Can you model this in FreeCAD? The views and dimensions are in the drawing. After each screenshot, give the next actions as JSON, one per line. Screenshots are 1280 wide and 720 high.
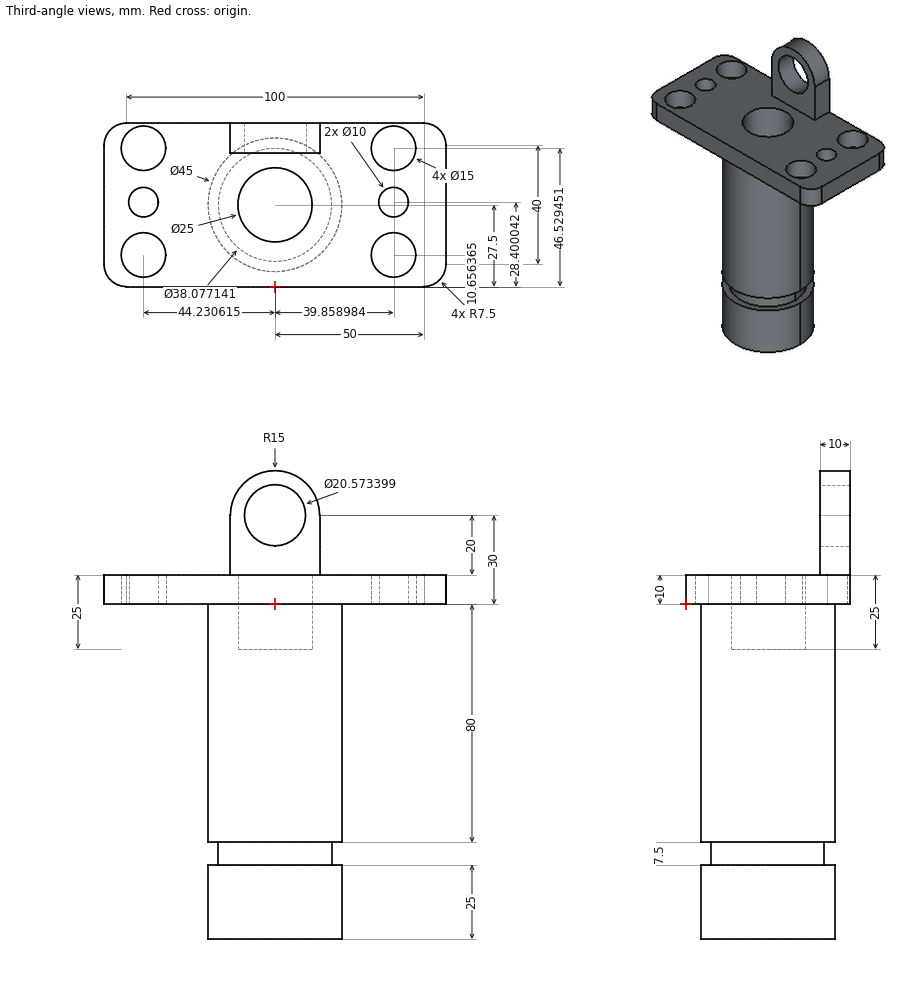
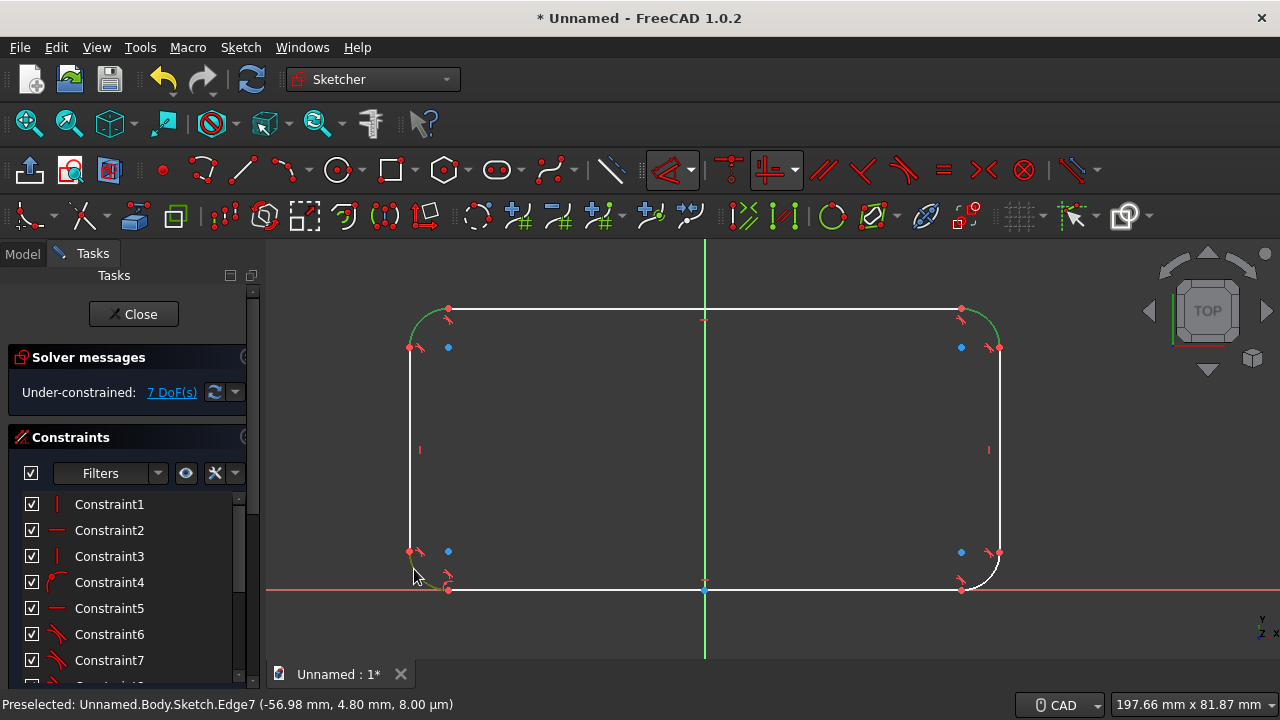
{"action": "left_click", "coordinate": [996, 570]}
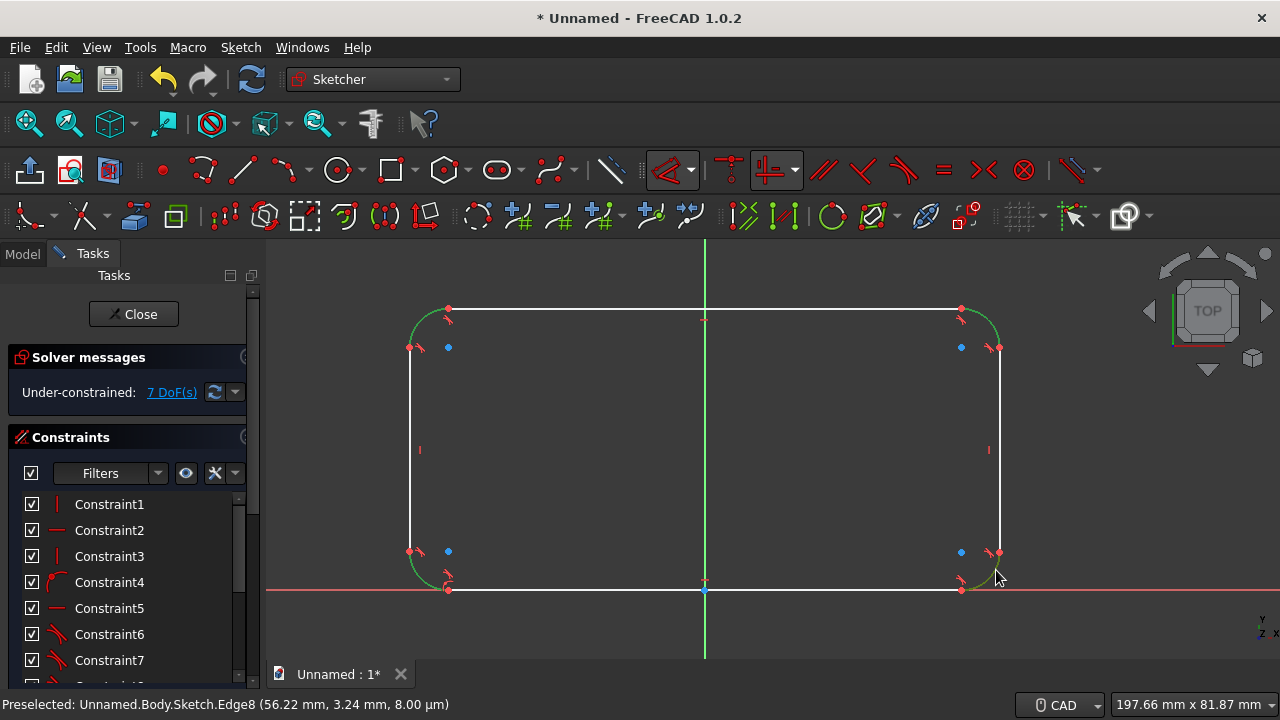
{"action": "left_click", "coordinate": [944, 170]}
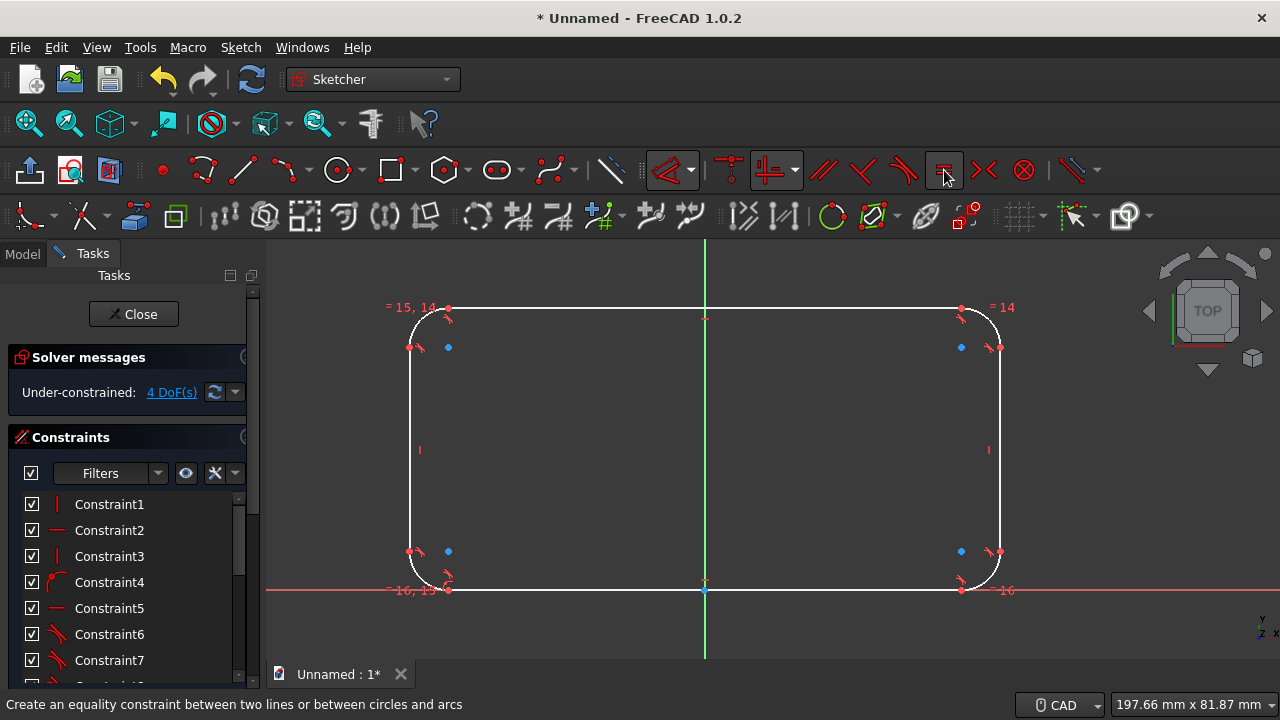
{"action": "left_click", "coordinate": [666, 170]}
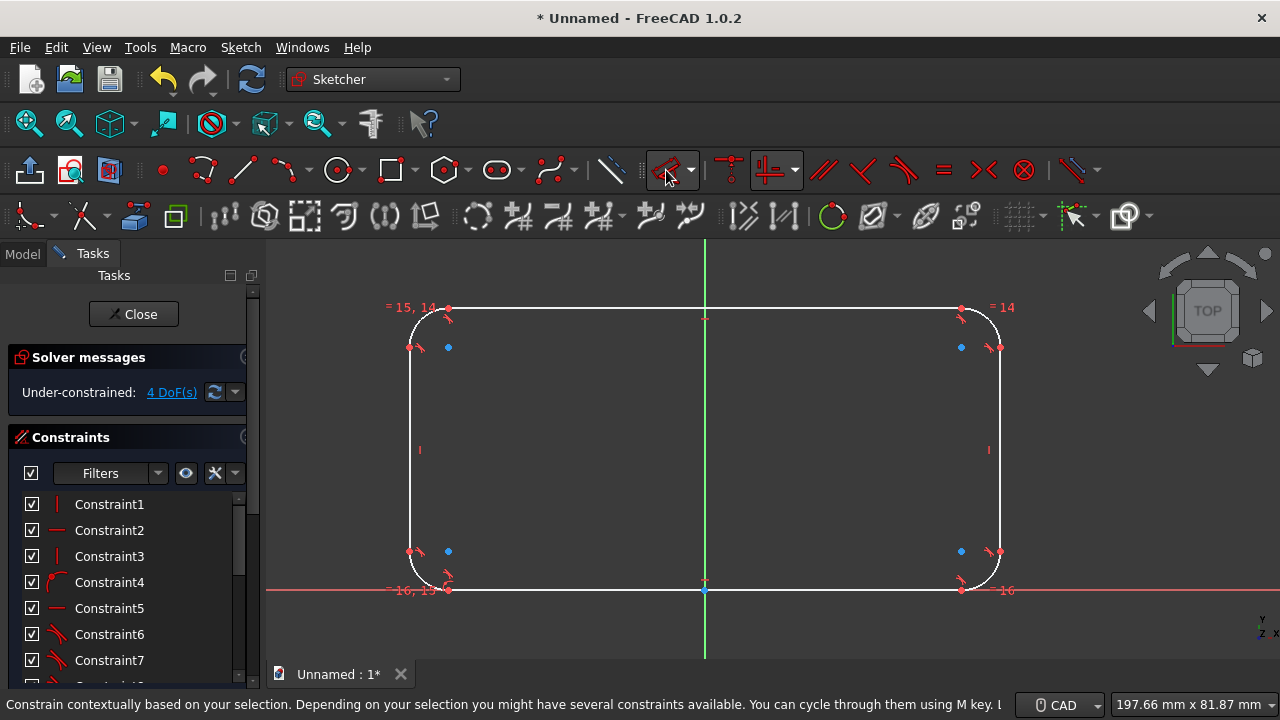
{"action": "left_click", "coordinate": [996, 330]}
{"action": "left_click", "coordinate": [1025, 316]}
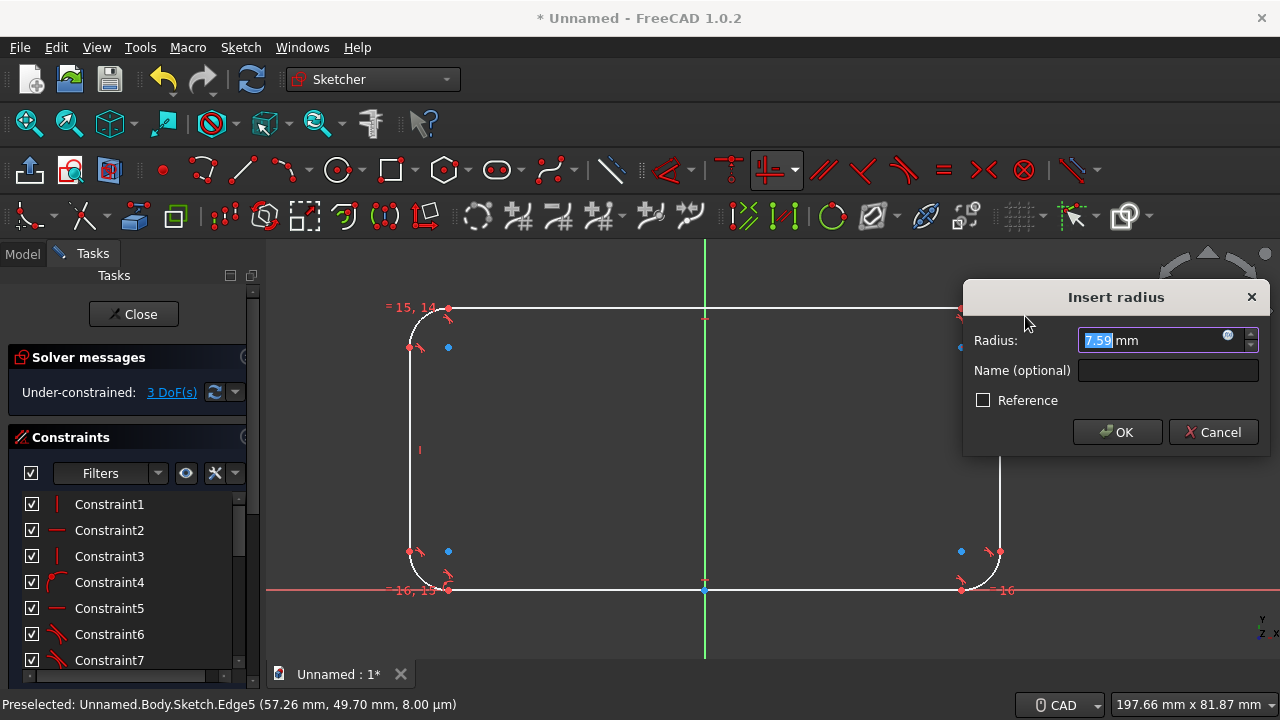
{"action": "type", "text": "7.5"}
{"action": "key", "text": "Return"}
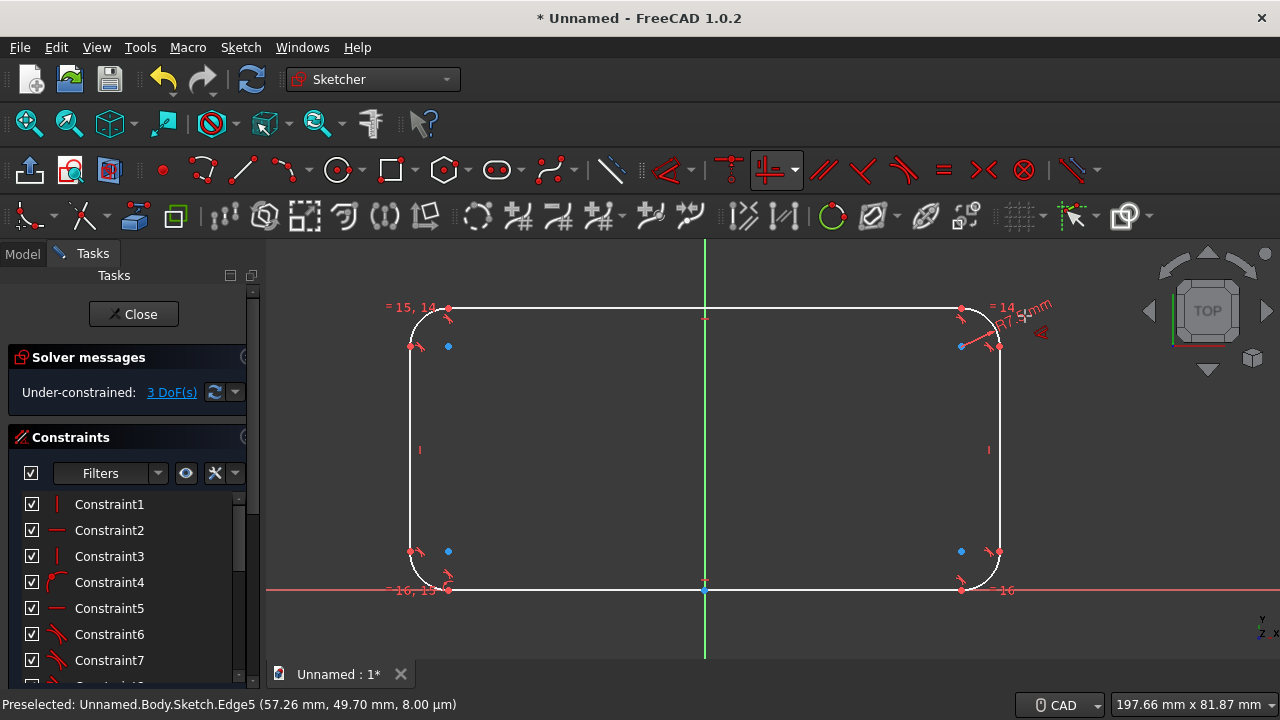
{"action": "left_click", "coordinate": [1000, 490]}
{"action": "left_click", "coordinate": [1034, 449]}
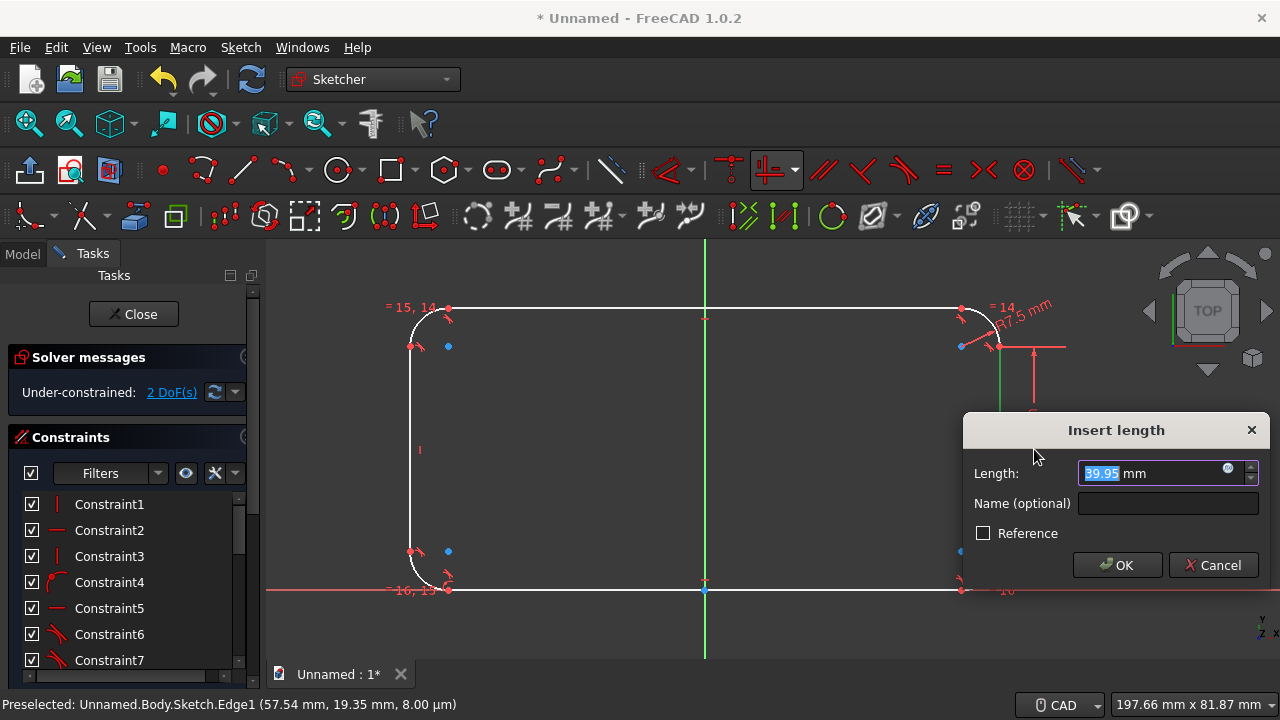
{"action": "type", "text": "40"}
{"action": "key", "text": "Return"}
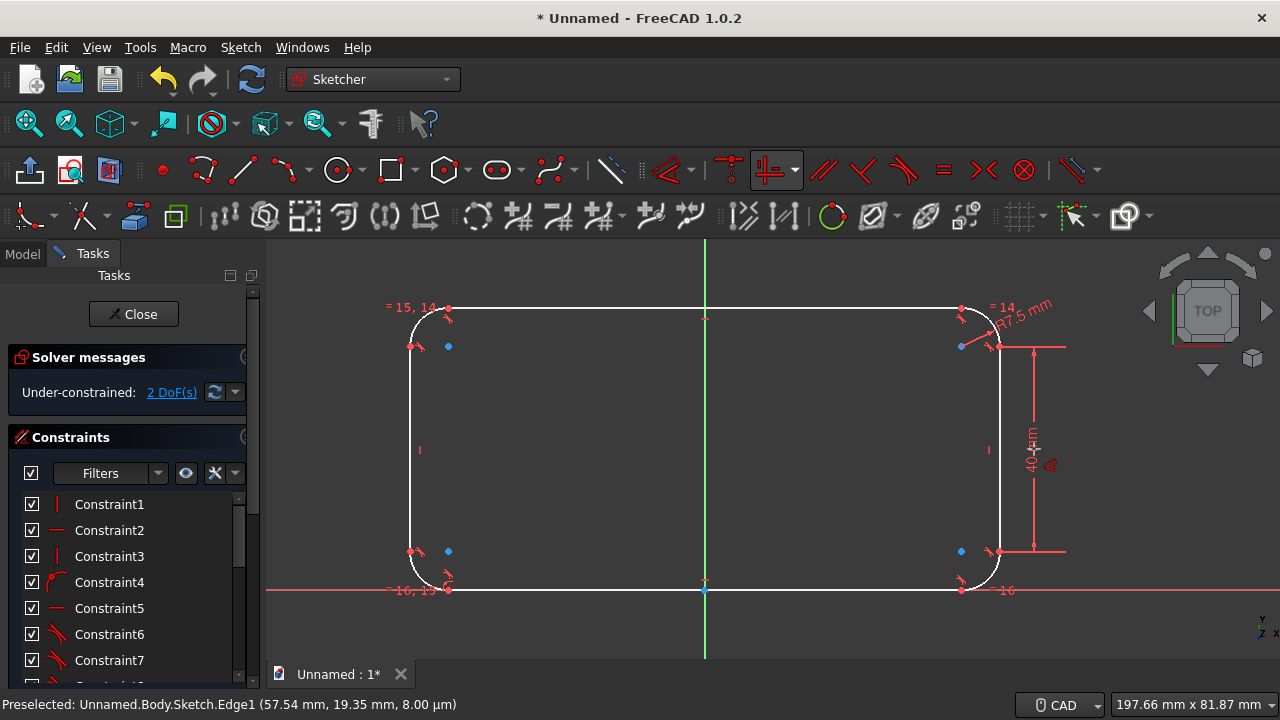
{"action": "left_click", "coordinate": [808, 308]}
{"action": "left_click", "coordinate": [587, 274]}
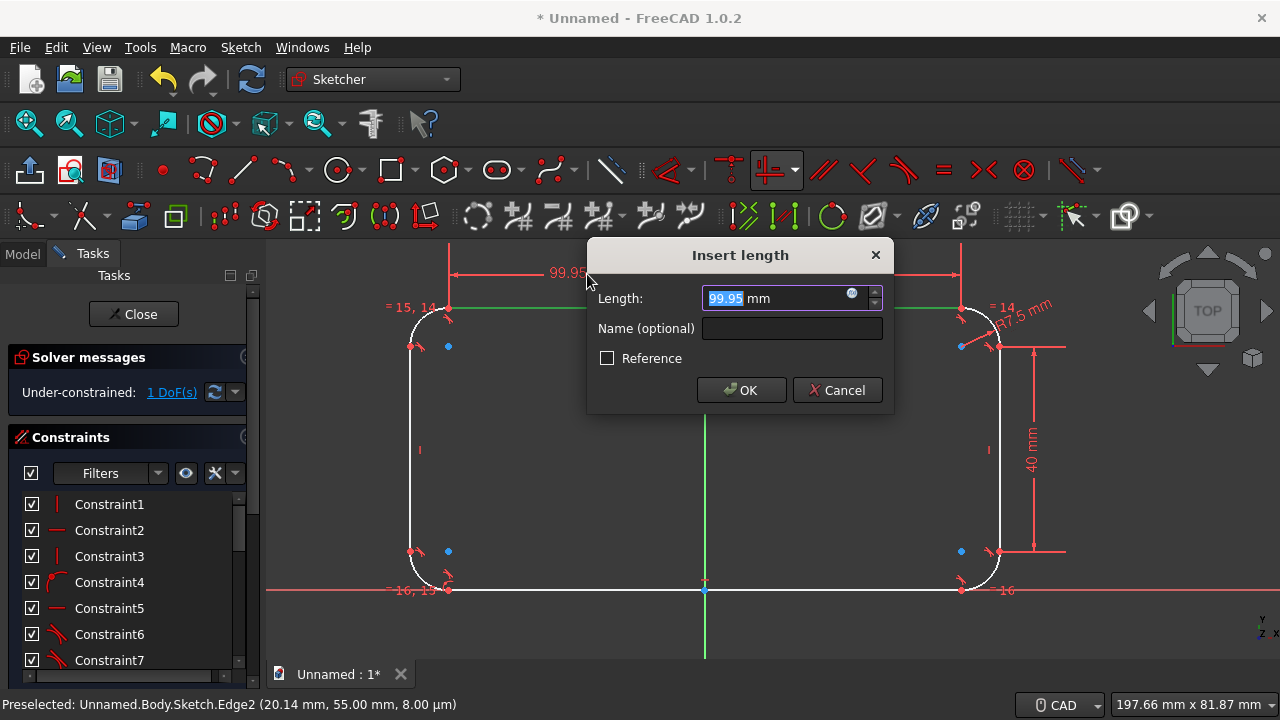
{"action": "type", "text": "100"}
{"action": "key", "text": "Return"}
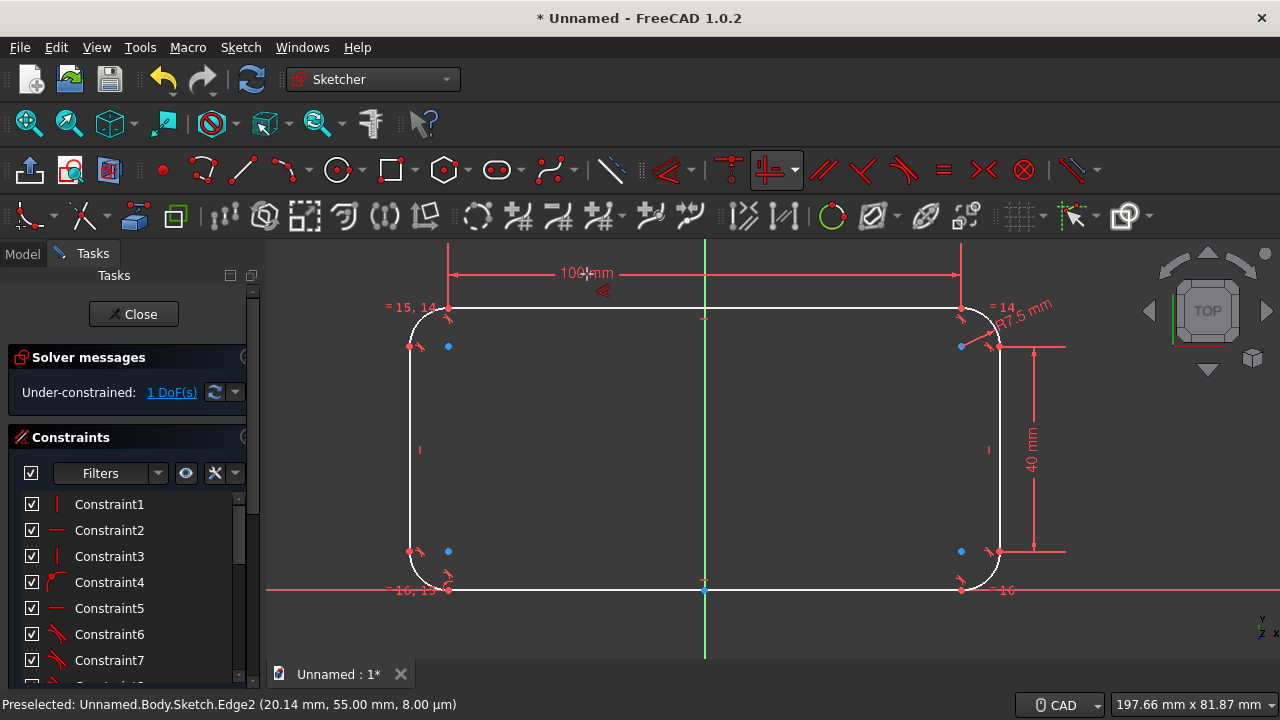
{"action": "left_click", "coordinate": [961, 308]}
{"action": "left_click", "coordinate": [833, 624]}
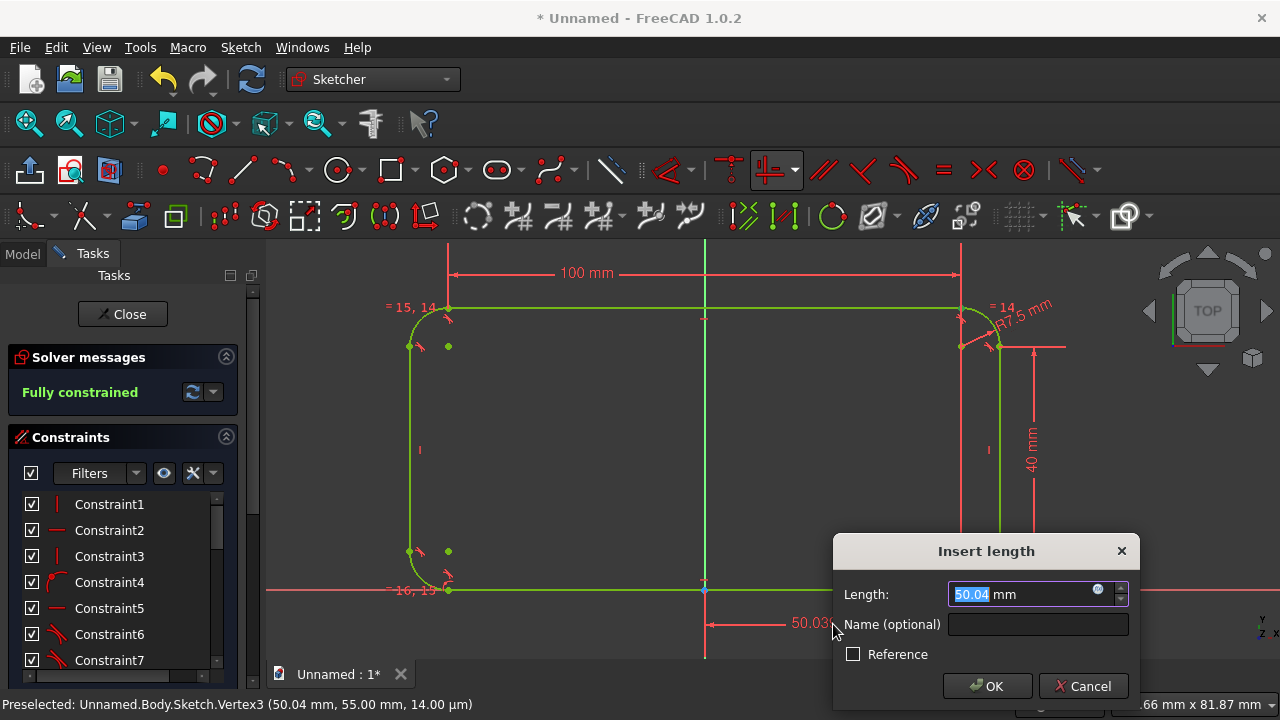
{"action": "type", "text": "50"}
{"action": "key", "text": "Return"}
{"action": "key", "text": "Escape"}